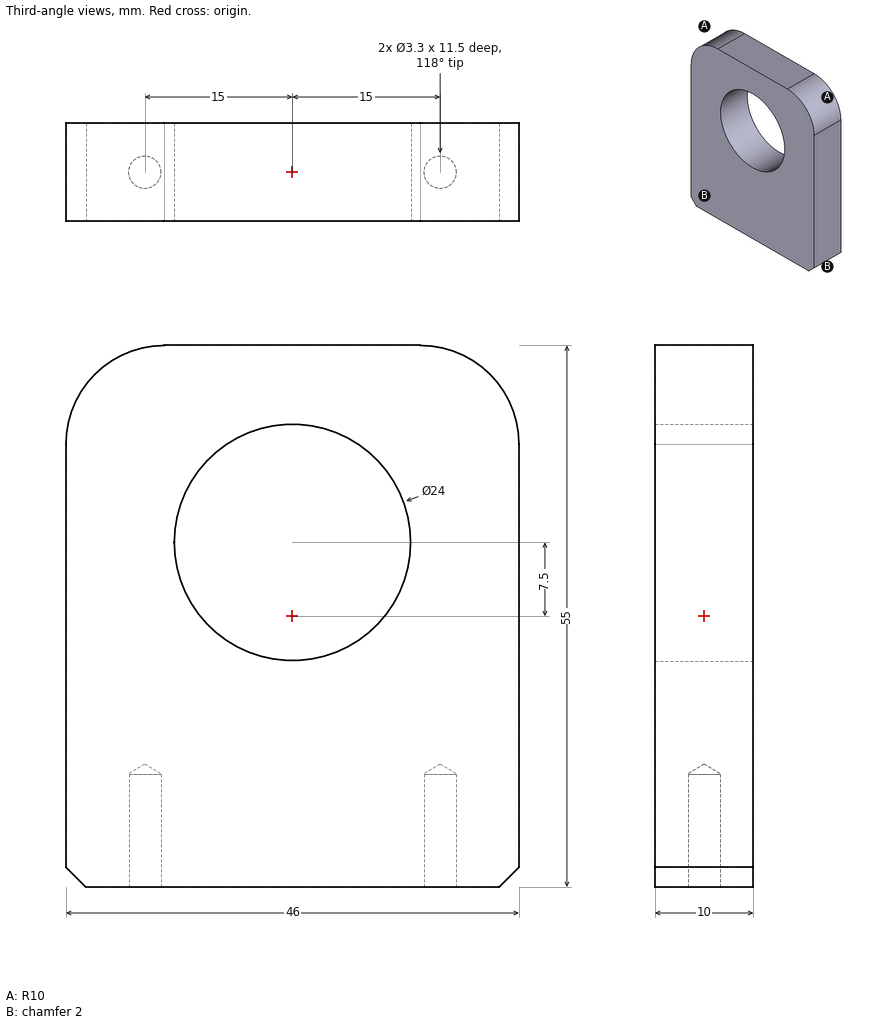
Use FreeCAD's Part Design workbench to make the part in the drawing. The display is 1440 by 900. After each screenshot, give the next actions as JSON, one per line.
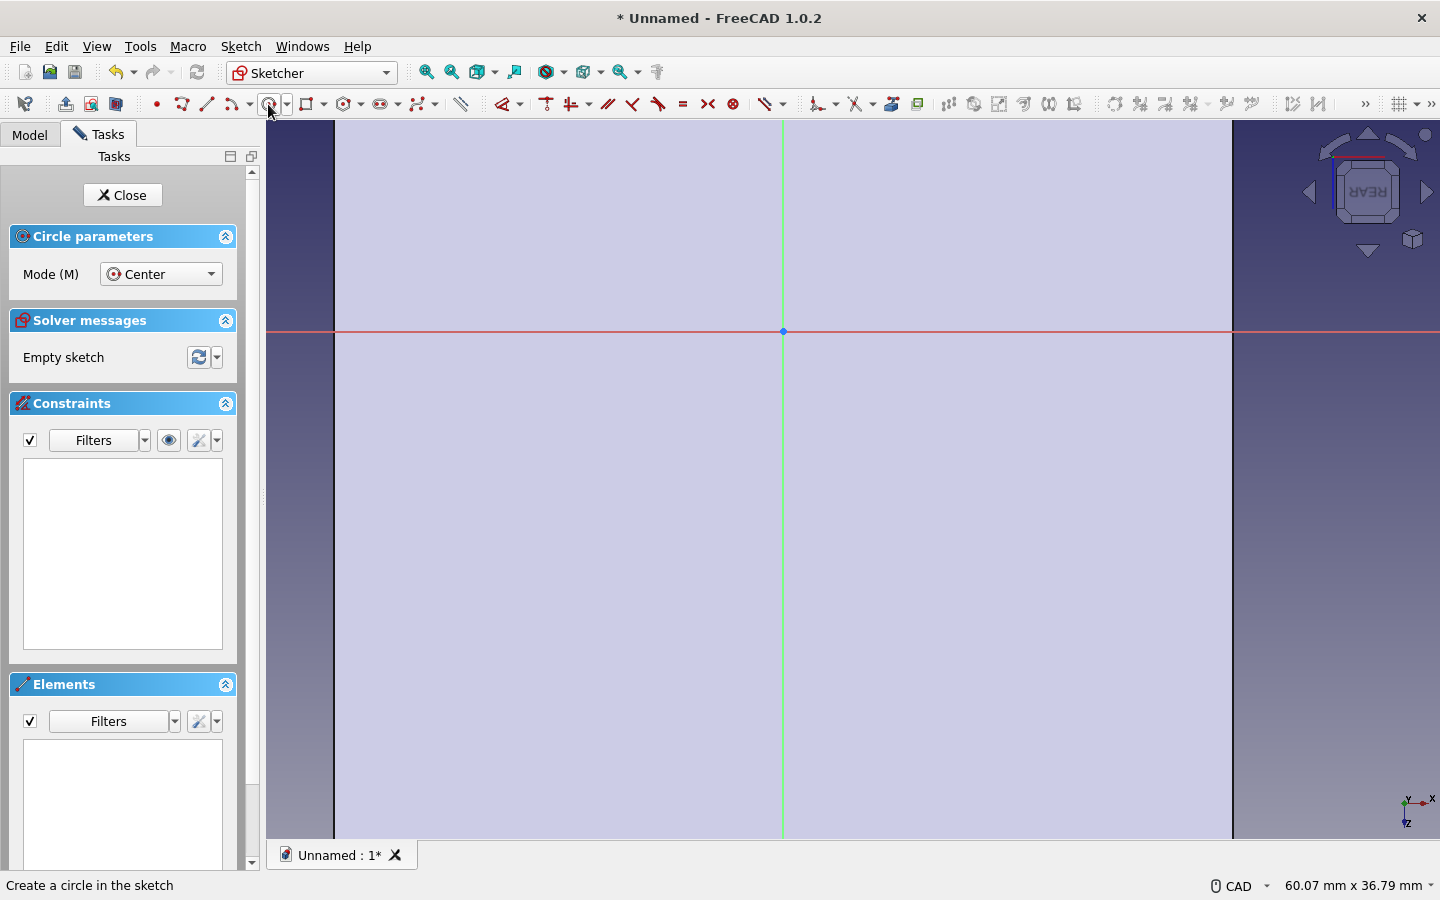
{"action": "left_click", "coordinate": [783, 478]}
{"action": "left_click", "coordinate": [949, 312]}
{"action": "key", "text": "Escape"}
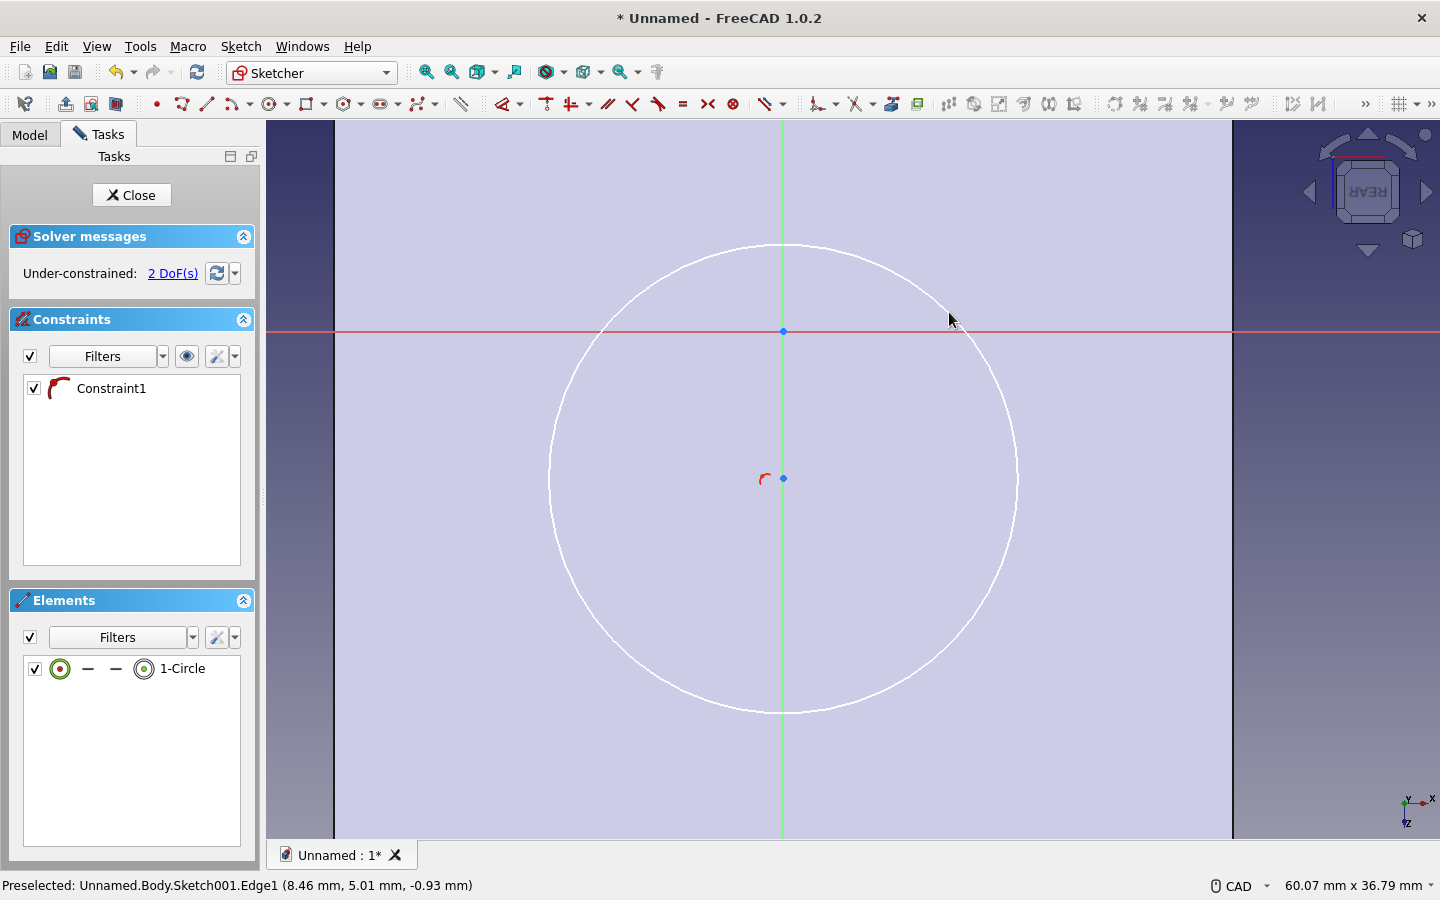
{"action": "key", "text": "d"}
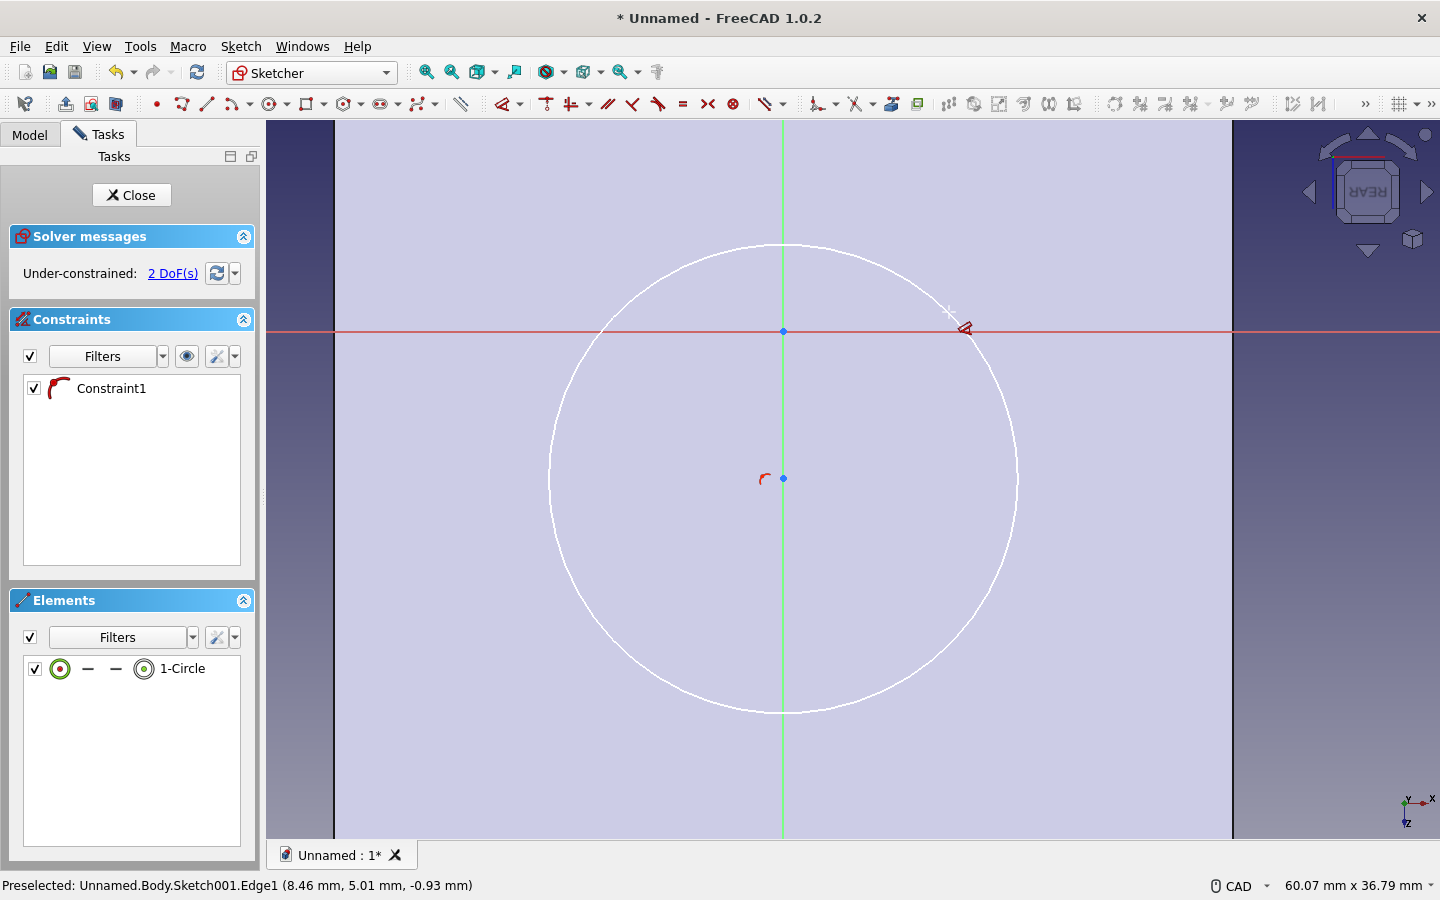
{"action": "left_click", "coordinate": [949, 313]}
{"action": "left_click", "coordinate": [972, 290]}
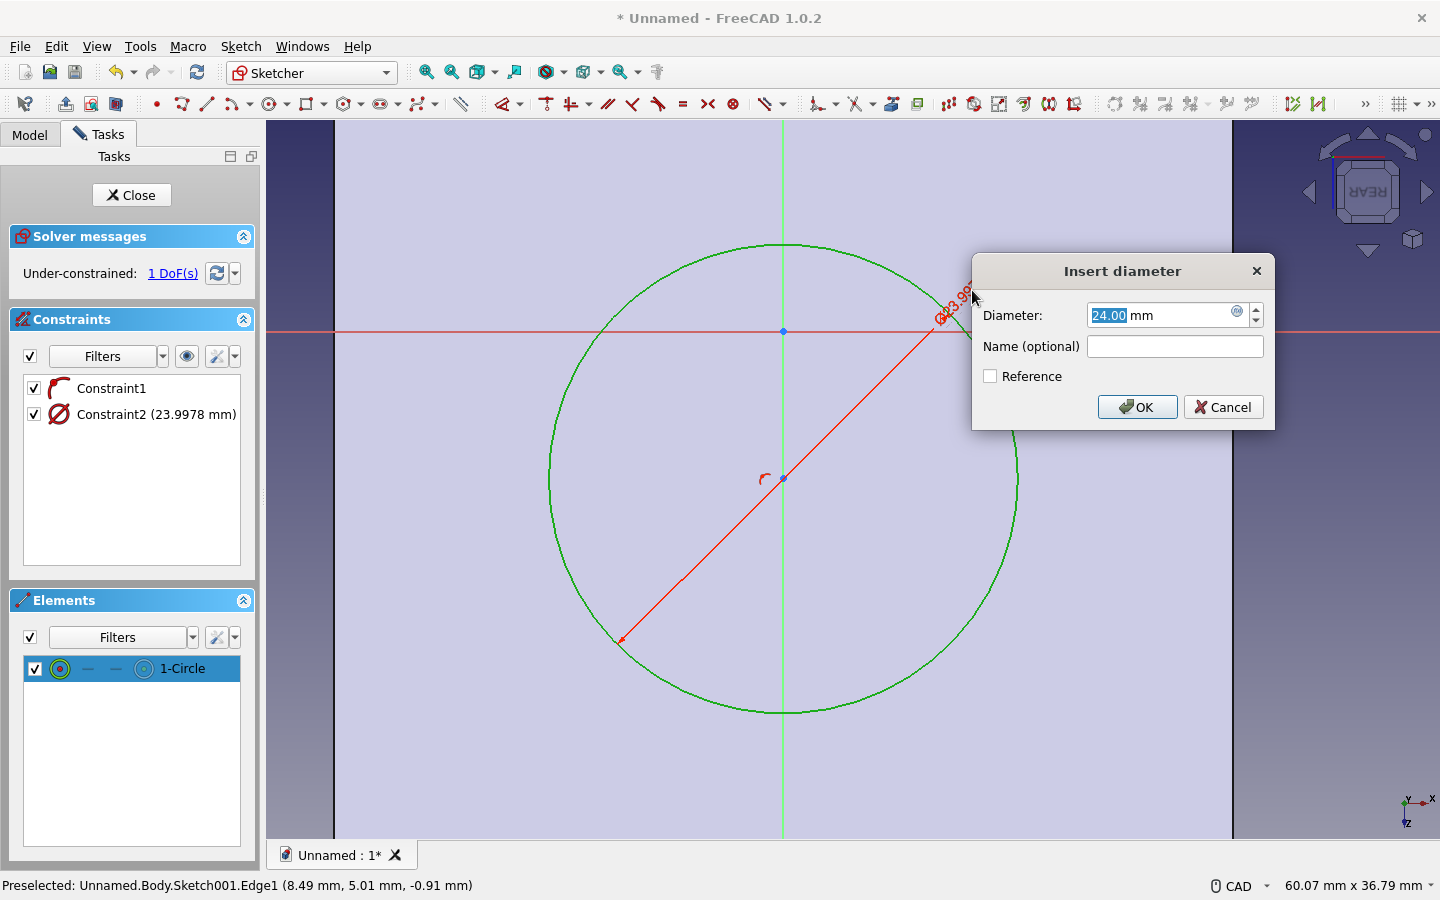
{"action": "type", "text": "24"}
{"action": "key", "text": "Return"}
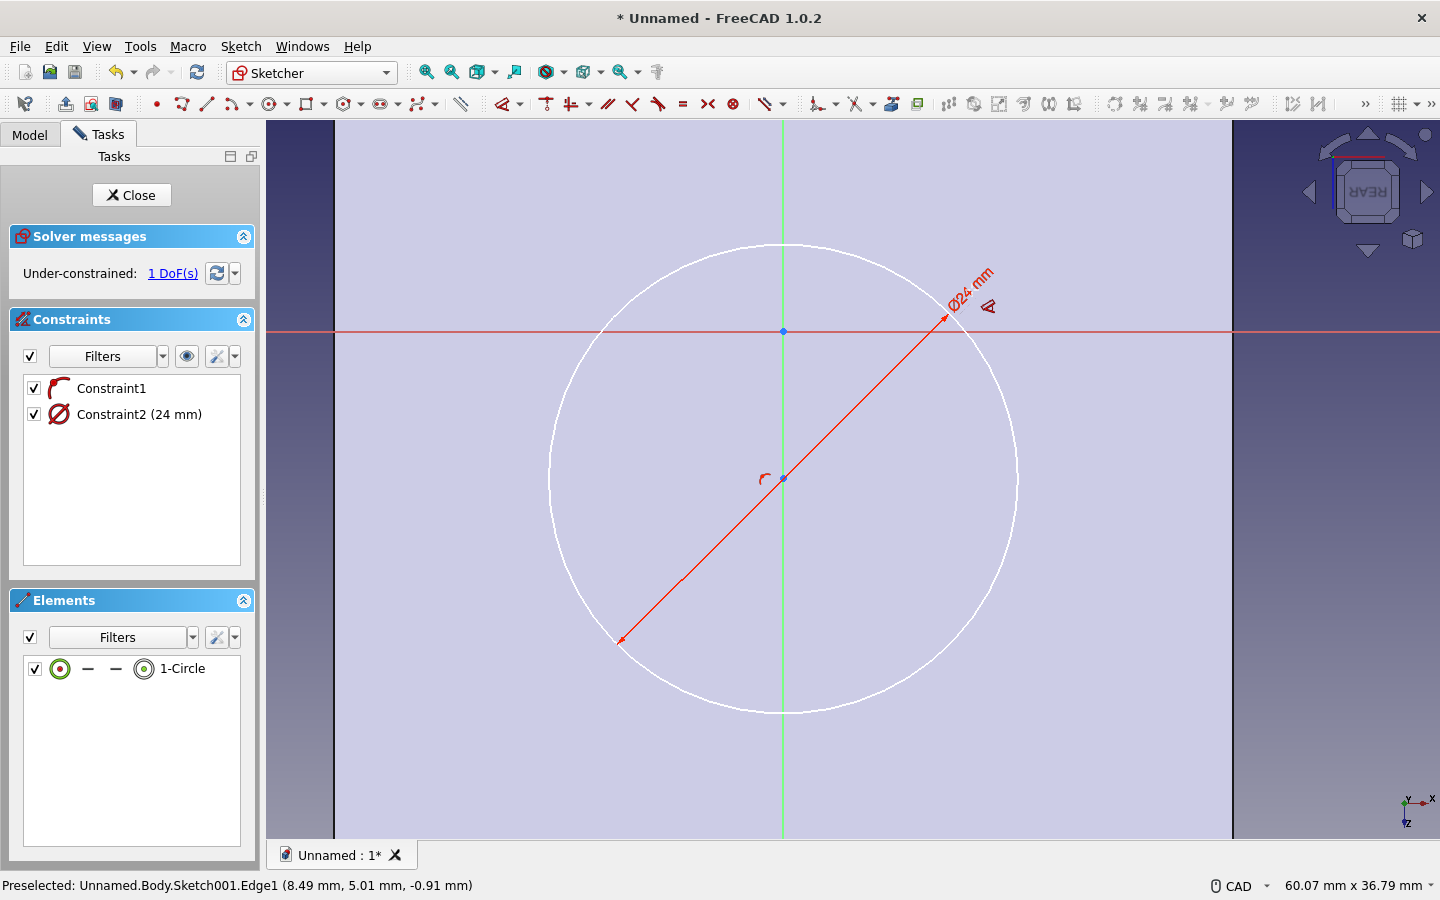
{"action": "left_click", "coordinate": [783, 479]}
{"action": "left_click", "coordinate": [817, 405]}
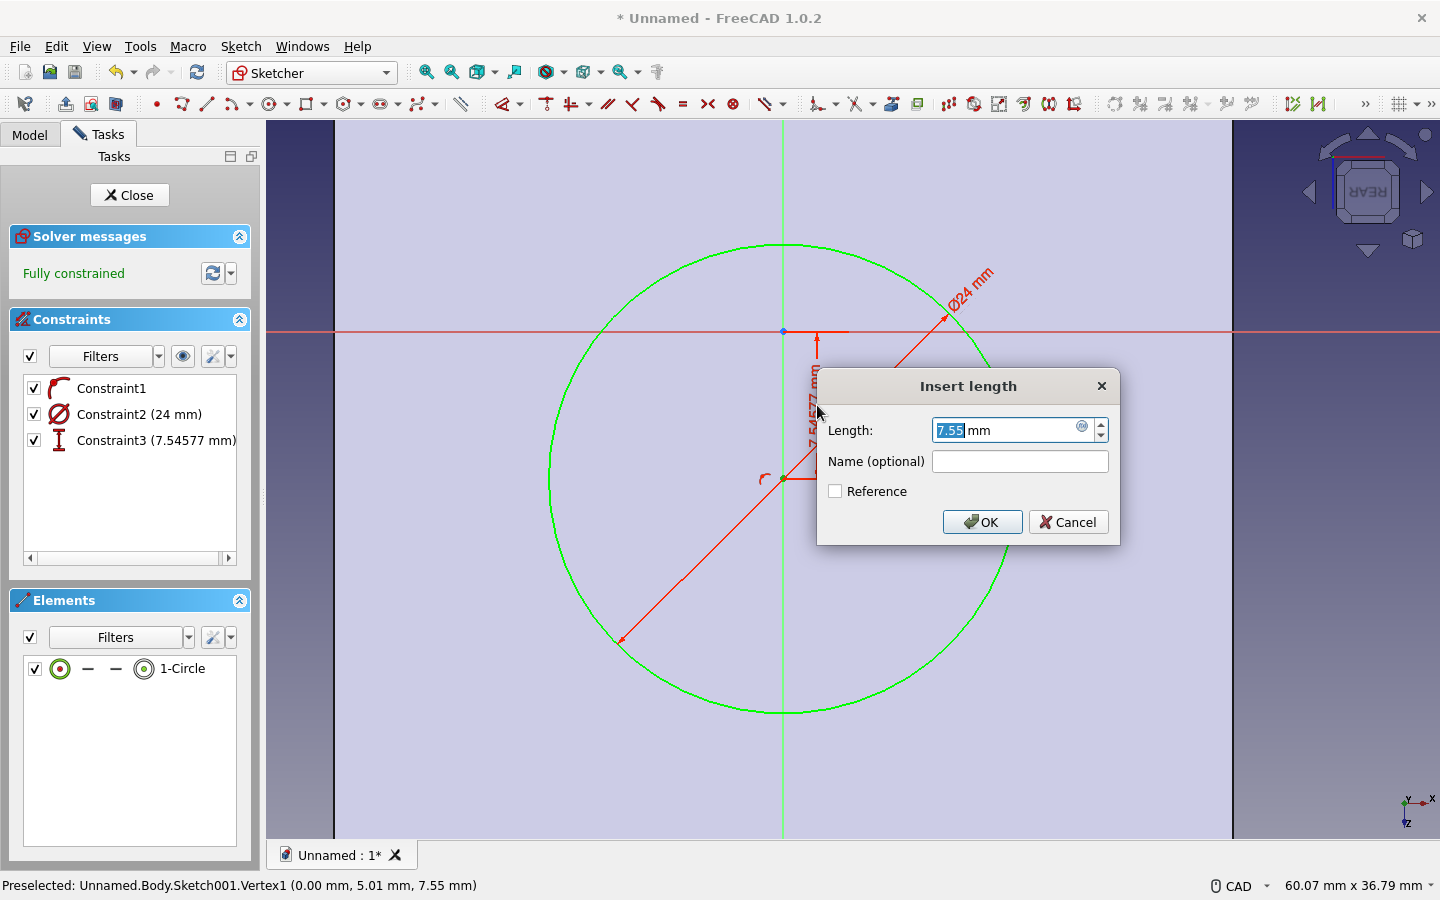
{"action": "type", "text": "7.5"}
{"action": "key", "text": "Return"}
{"action": "key", "text": "Escape"}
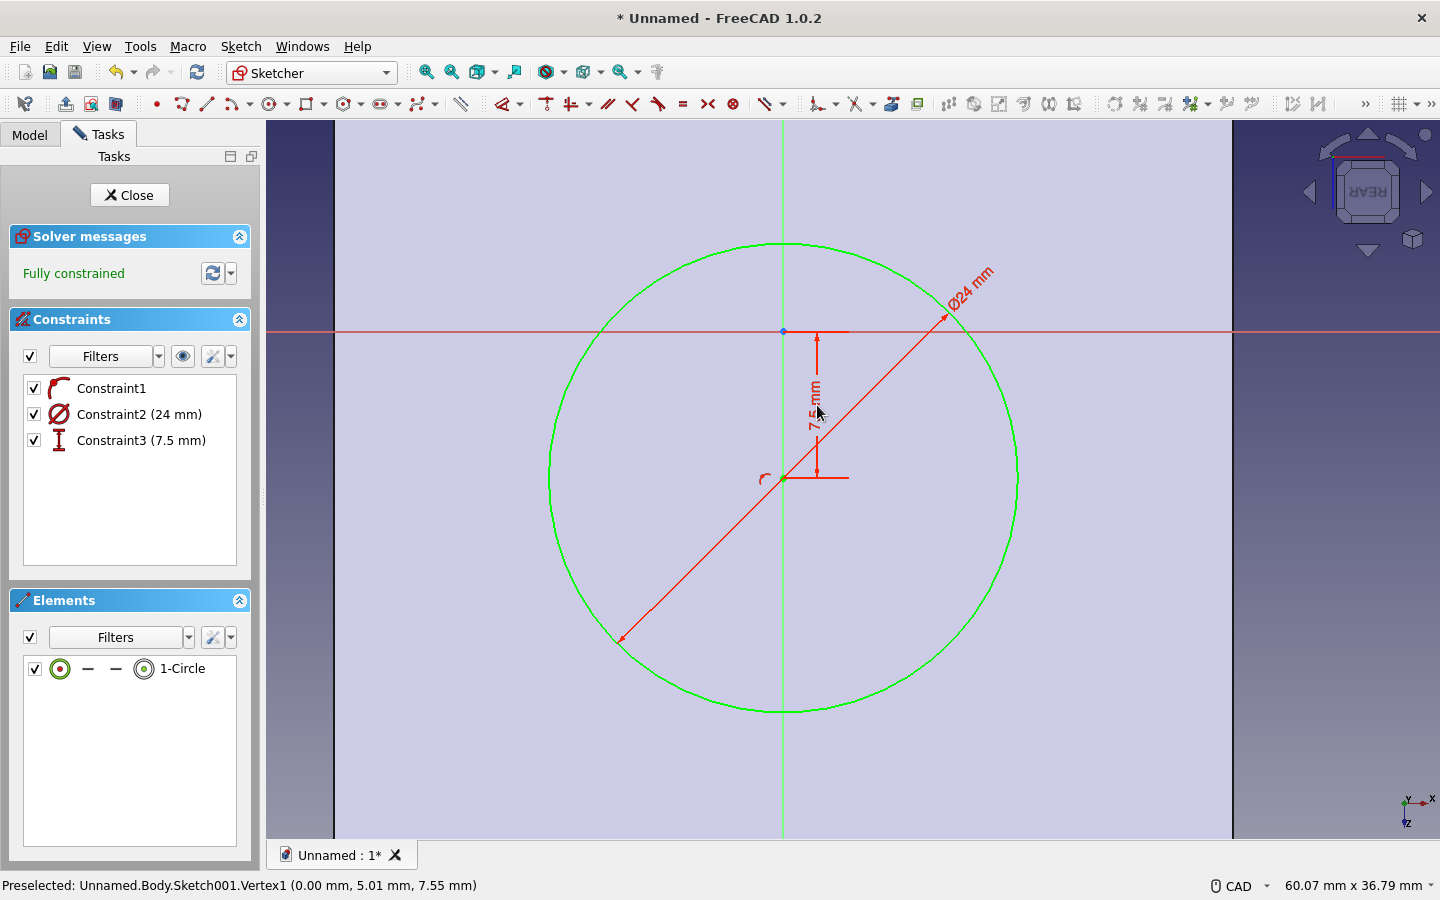
{"action": "left_click", "coordinate": [130, 195]}